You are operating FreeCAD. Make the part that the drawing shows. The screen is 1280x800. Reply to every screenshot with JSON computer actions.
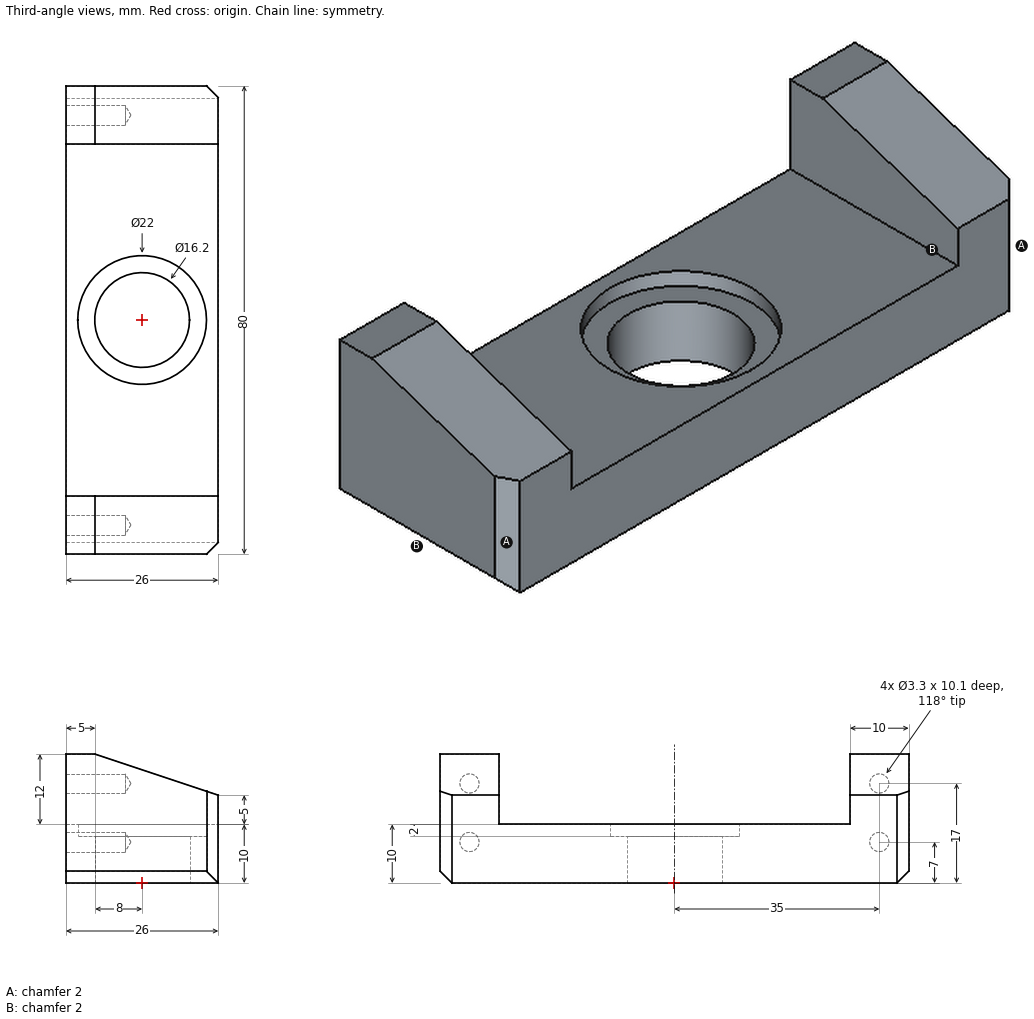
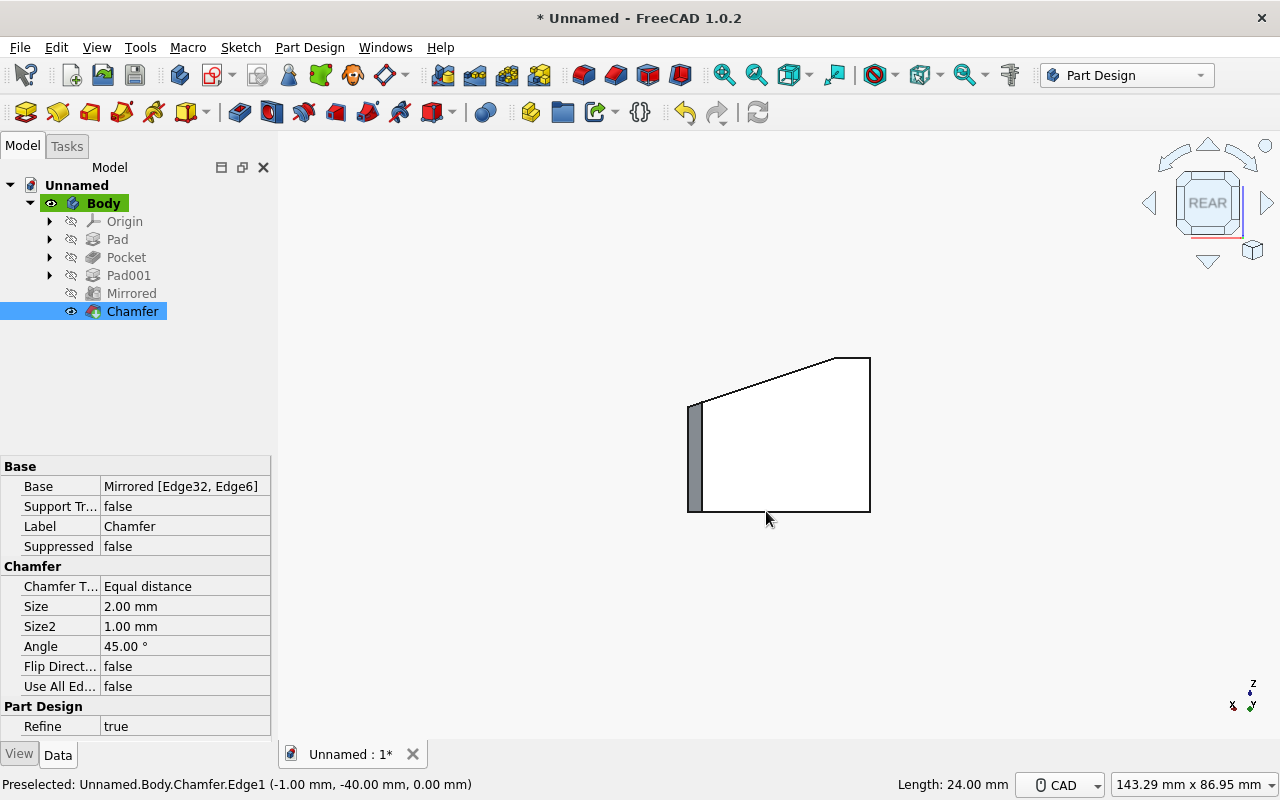
{"action": "left_click", "coordinate": [726, 76]}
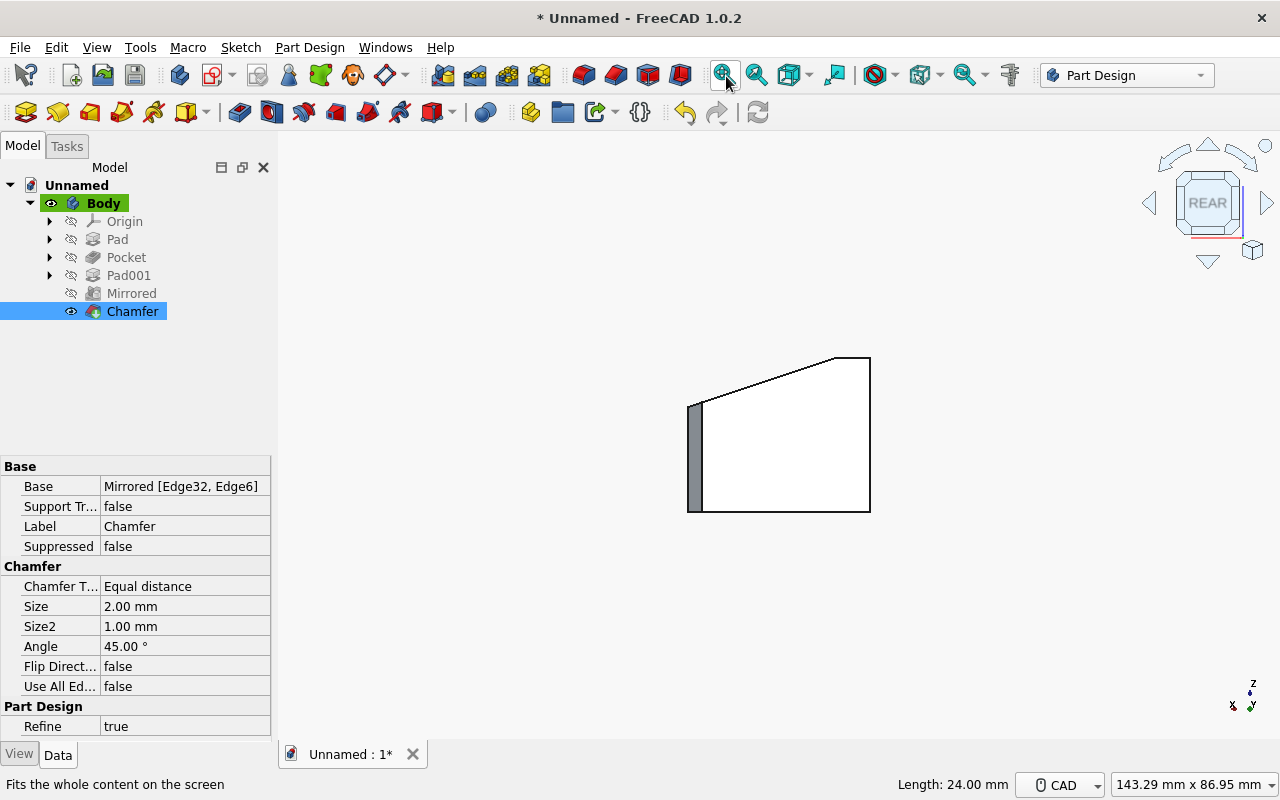
{"action": "left_click", "coordinate": [786, 511], "text": "ctrl"}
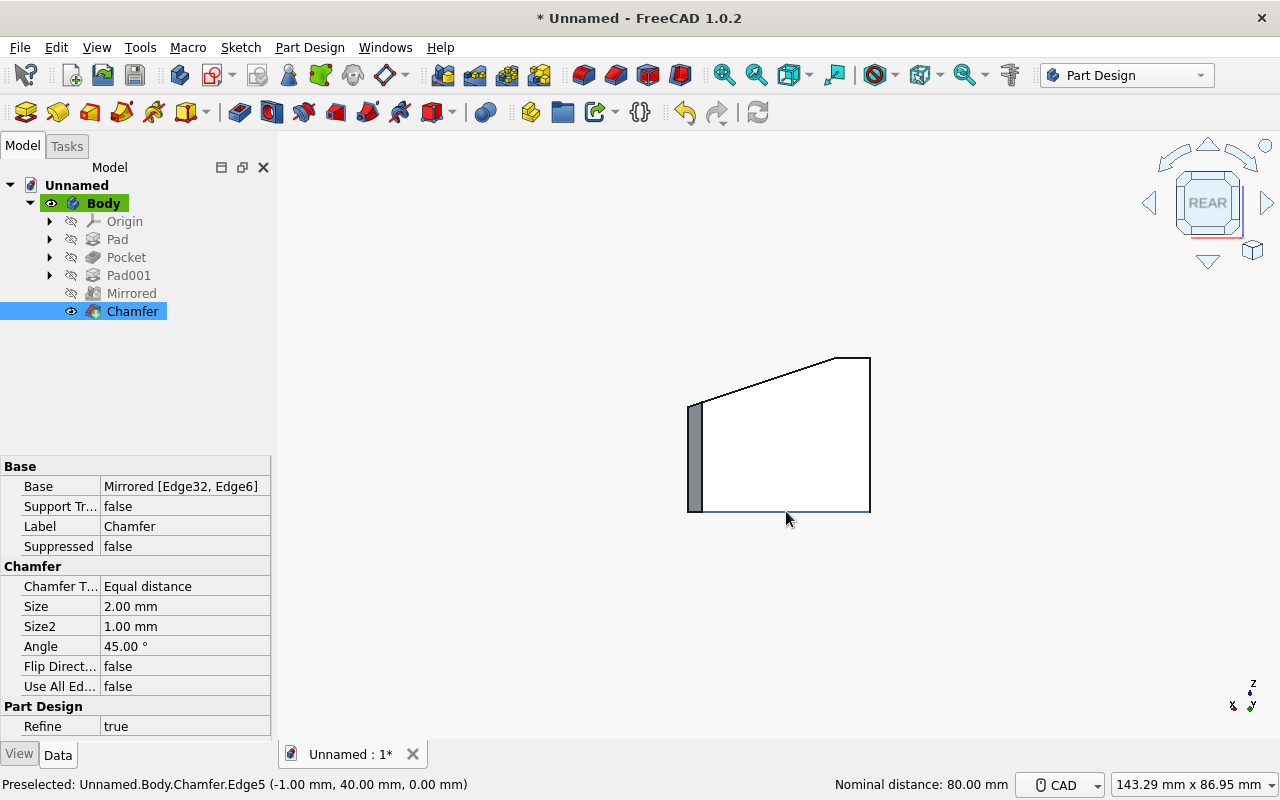
{"action": "left_click", "coordinate": [616, 76]}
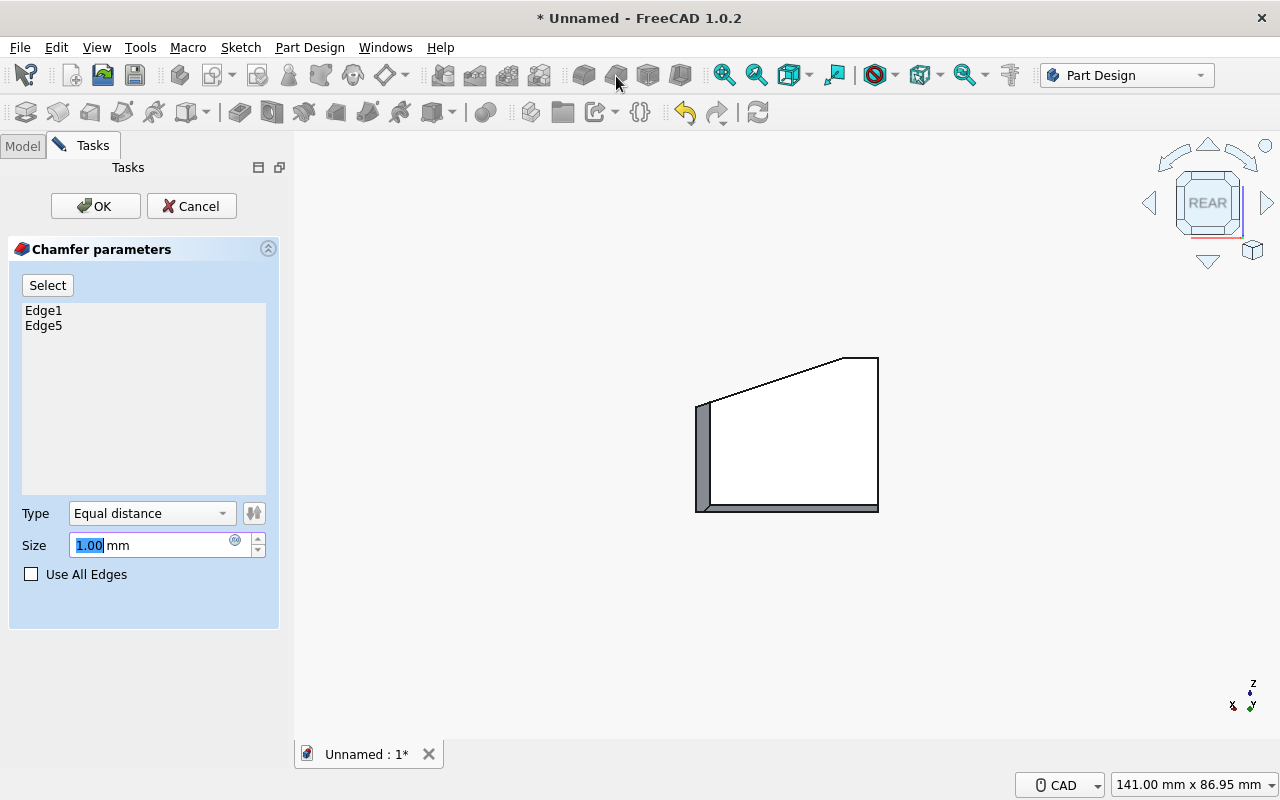
{"action": "type", "text": "2"}
{"action": "key", "text": "Tab"}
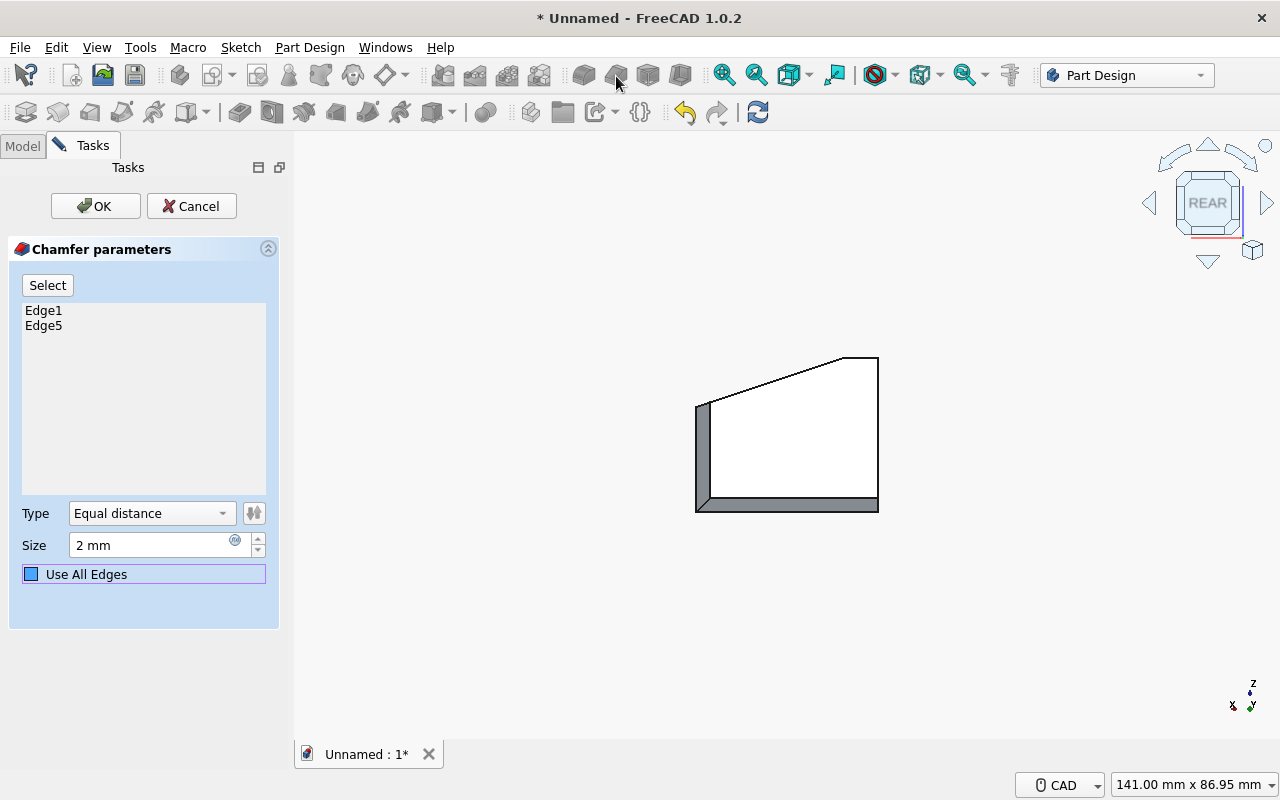
{"action": "left_click", "coordinate": [96, 206]}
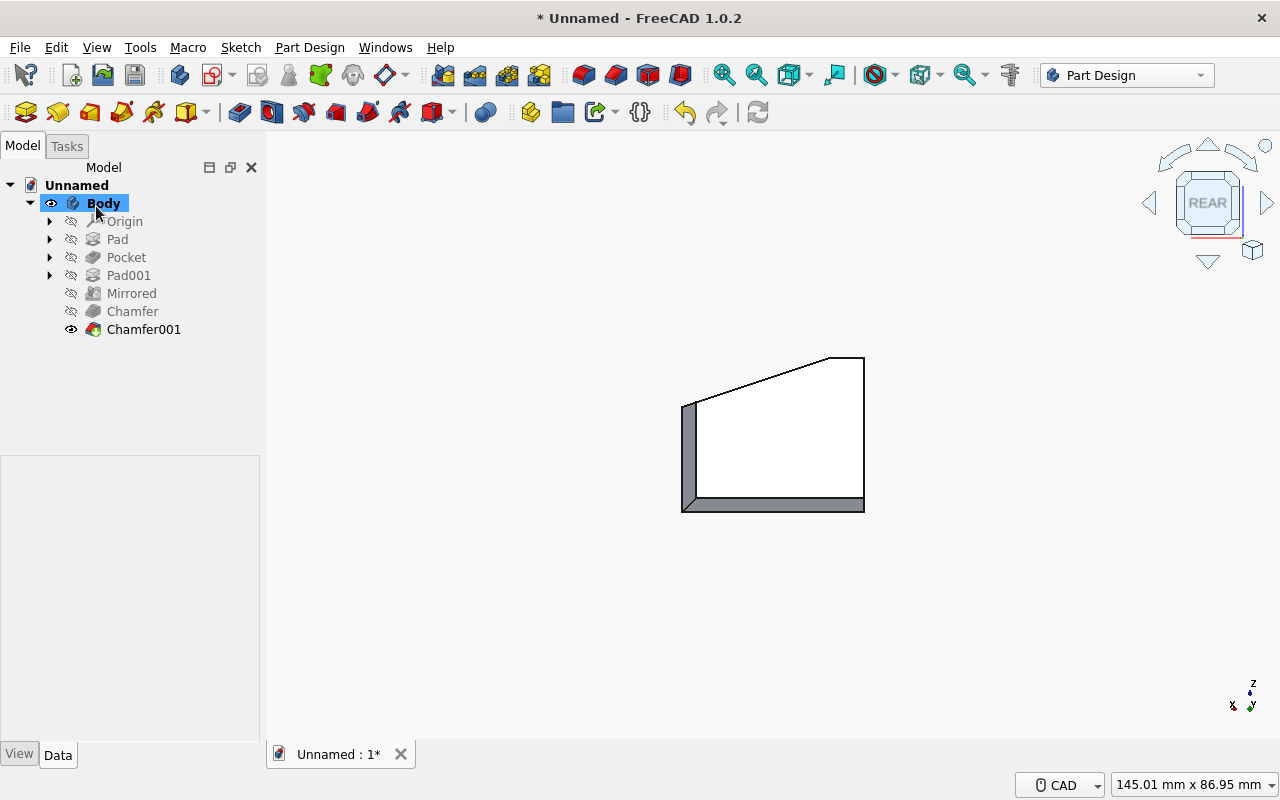
{"action": "left_click", "coordinate": [726, 76]}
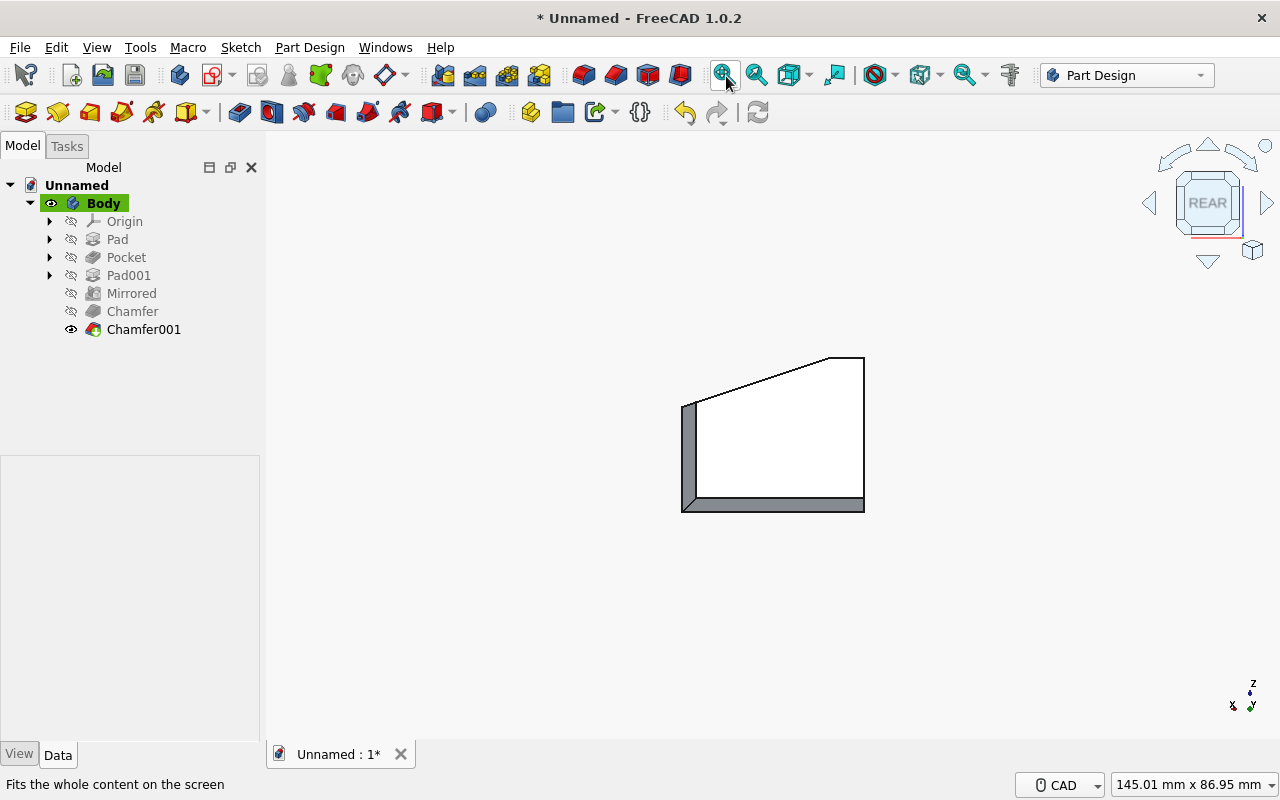
{"action": "key", "text": "0"}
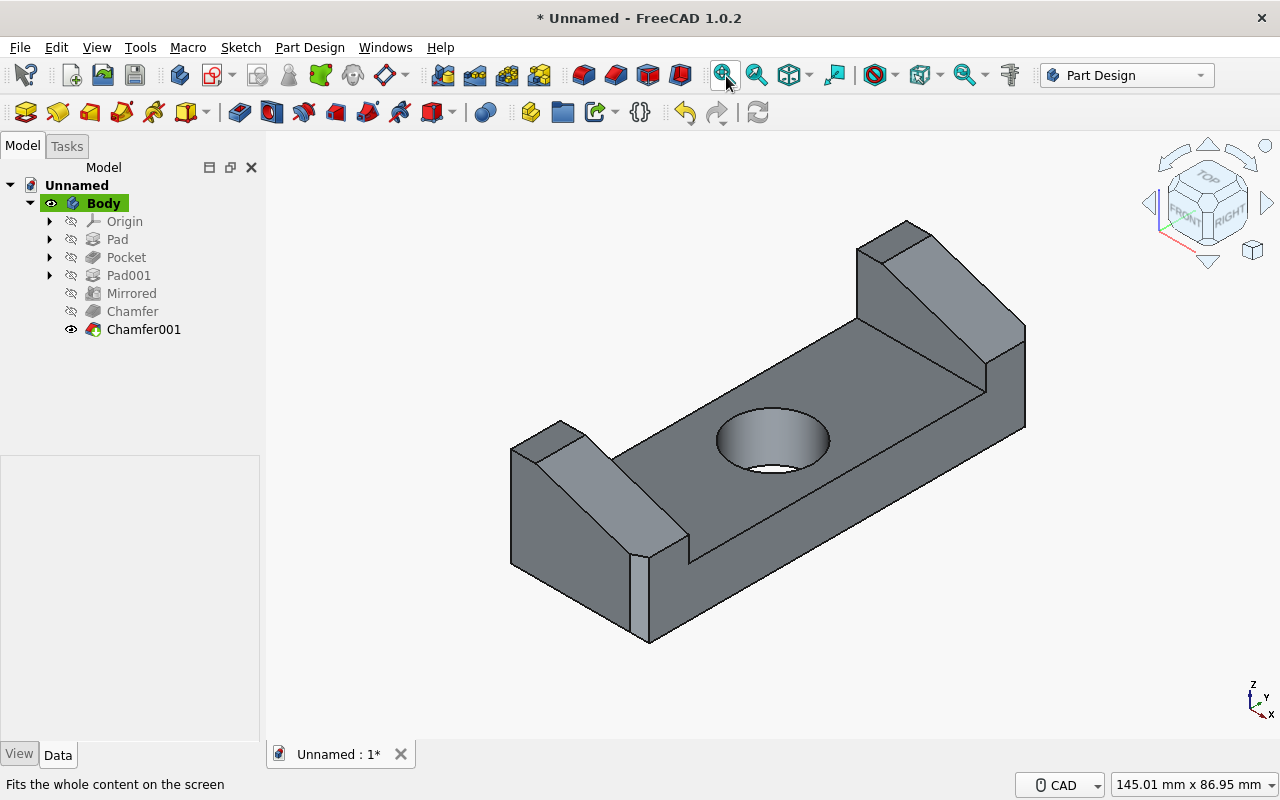
{"action": "left_click", "coordinate": [839, 380]}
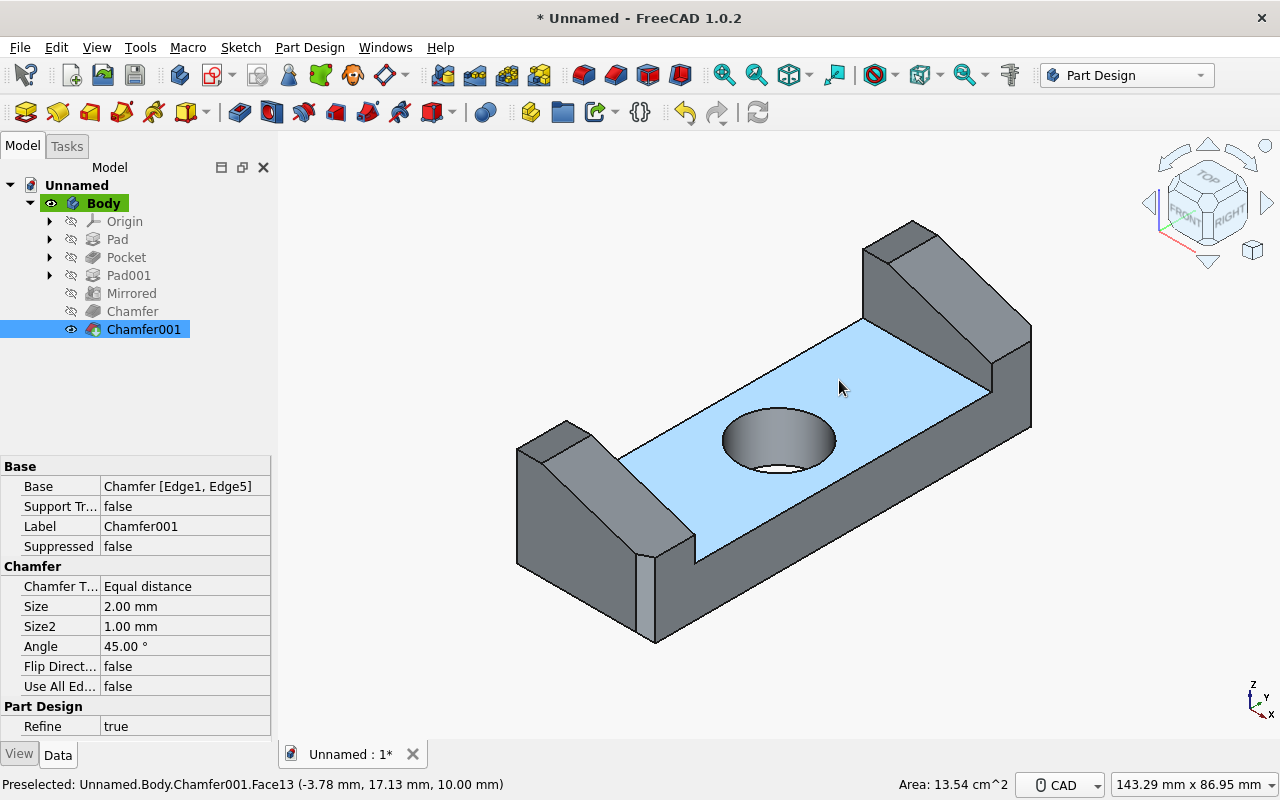
{"action": "left_click", "coordinate": [212, 76]}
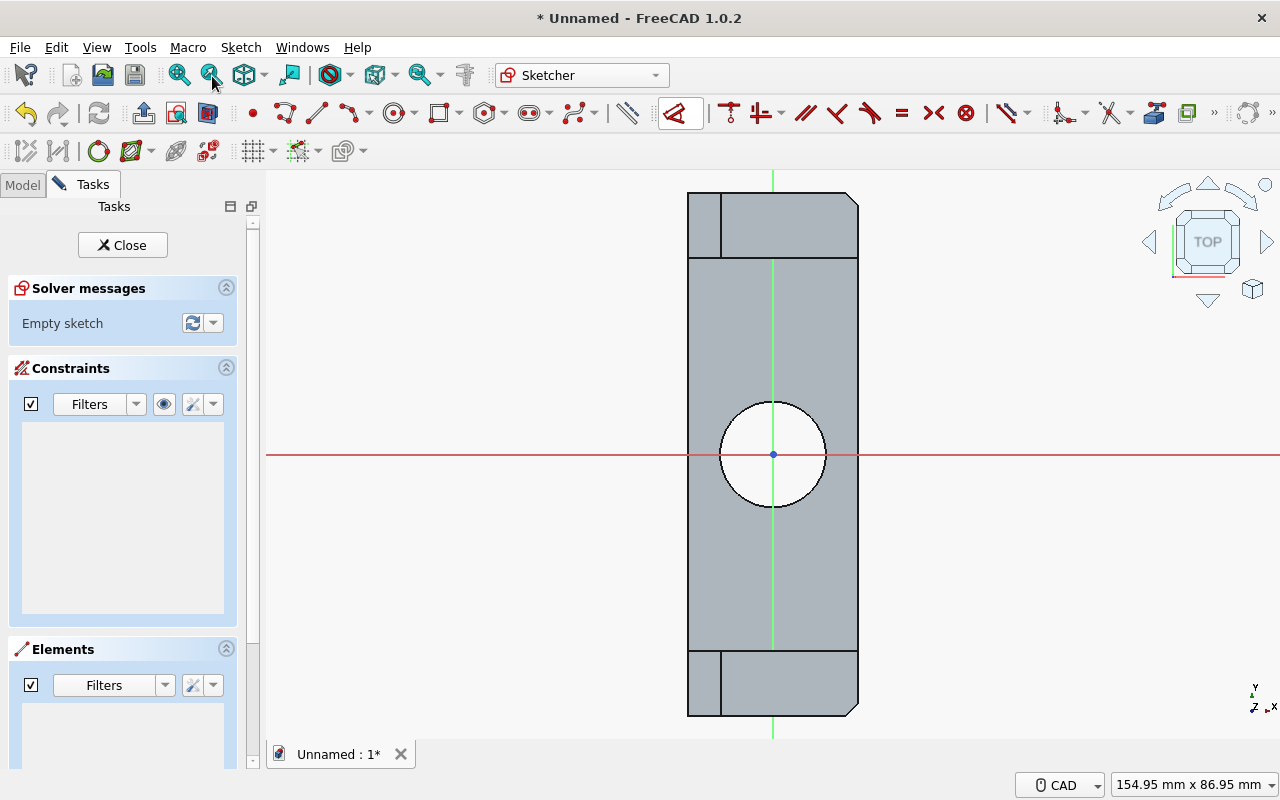
{"action": "scroll", "coordinate": [813, 454], "scroll_direction": "up", "scroll_amount": 5}